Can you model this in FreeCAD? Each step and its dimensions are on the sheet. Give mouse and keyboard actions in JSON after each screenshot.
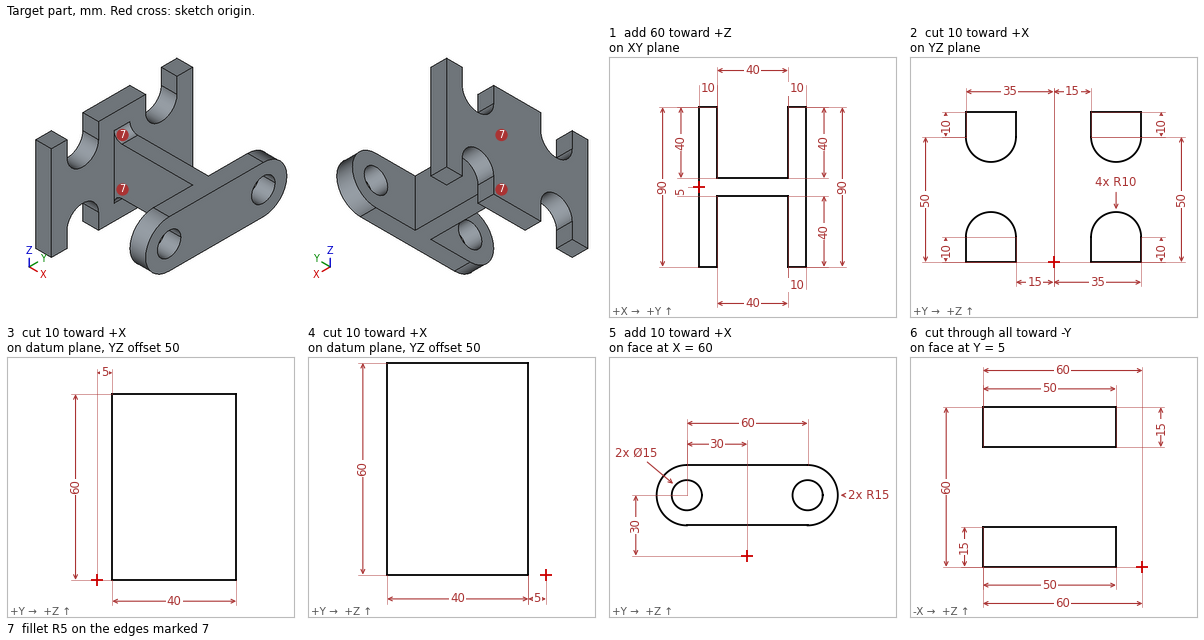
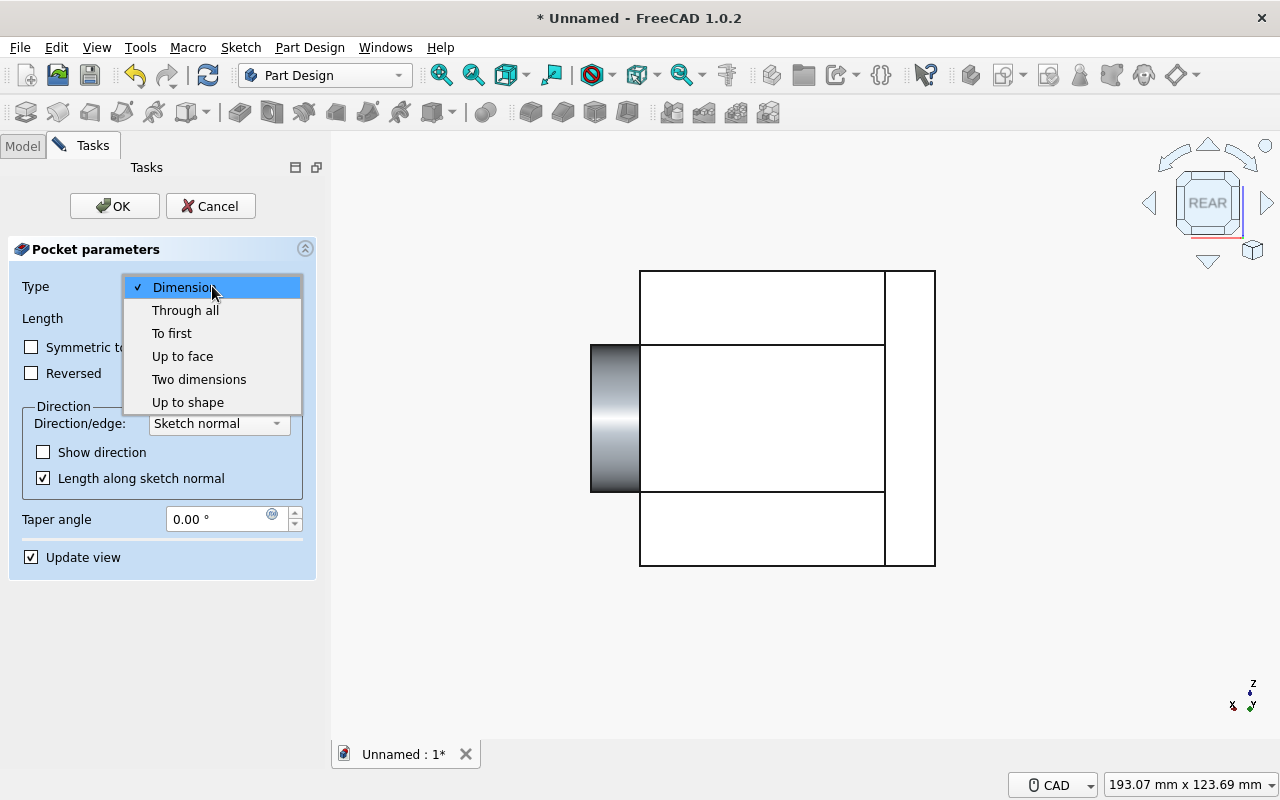
{"action": "left_click", "coordinate": [212, 310]}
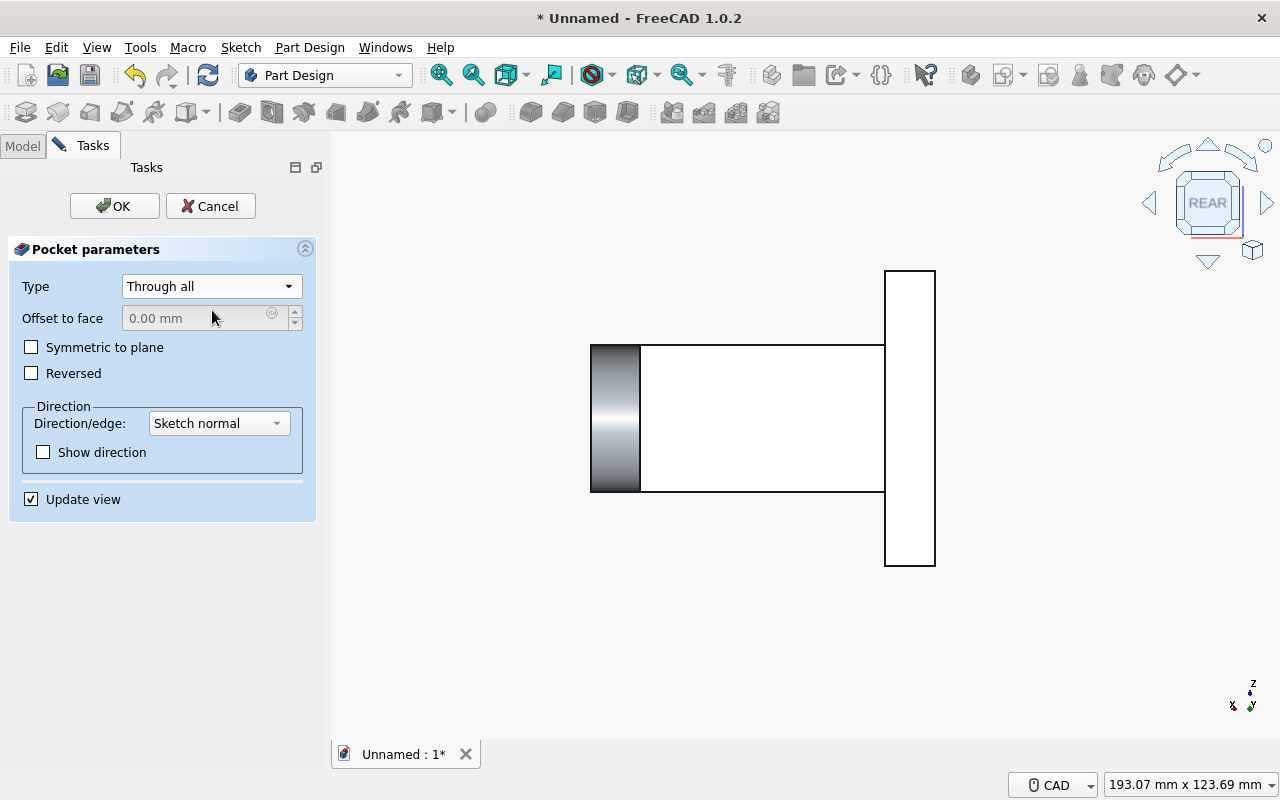
{"action": "left_click", "coordinate": [115, 206]}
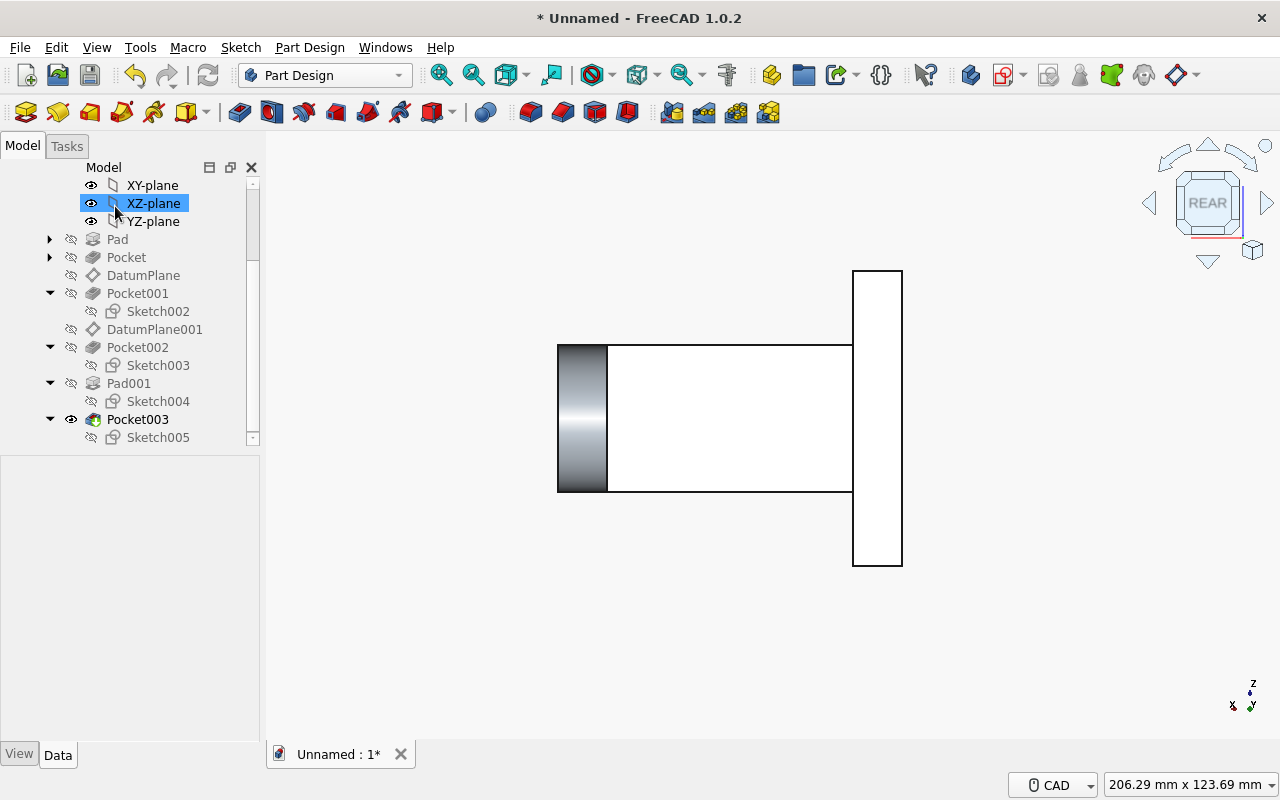
{"action": "key", "text": "0"}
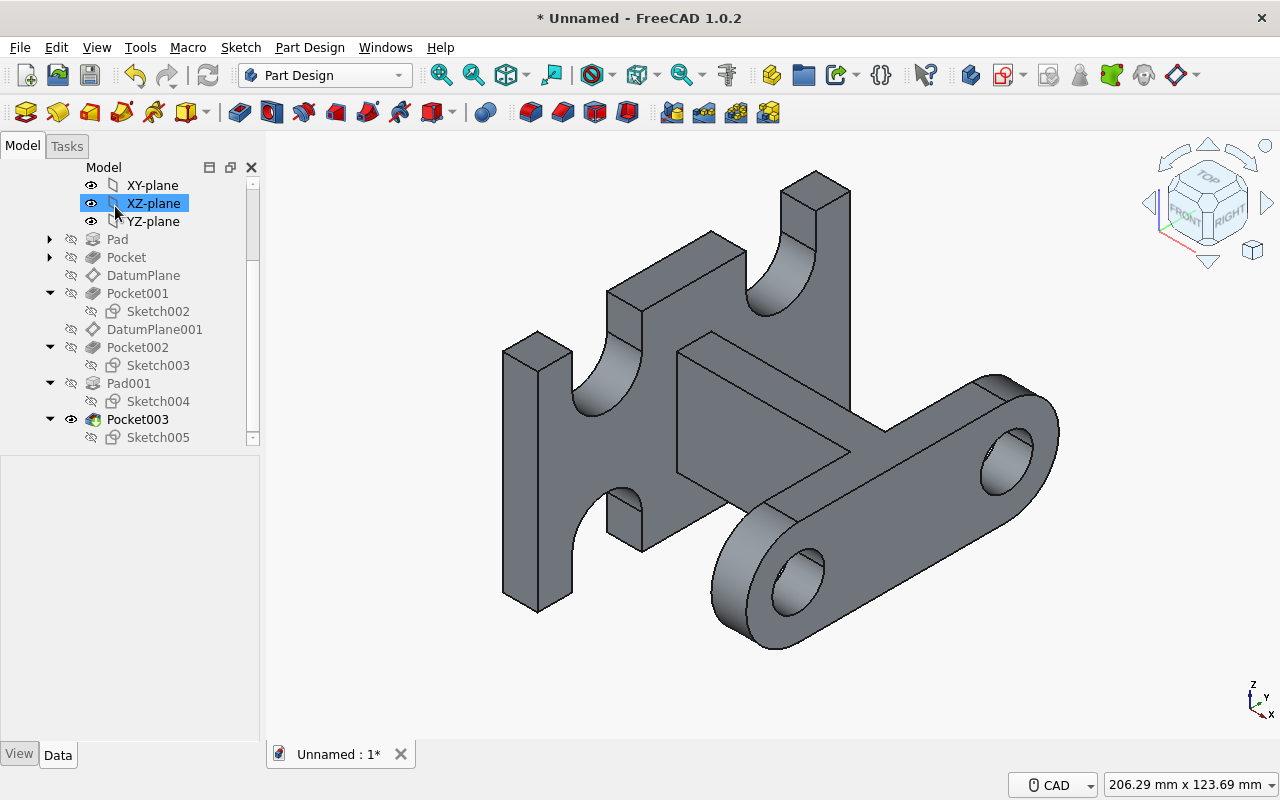
{"action": "key", "text": "2"}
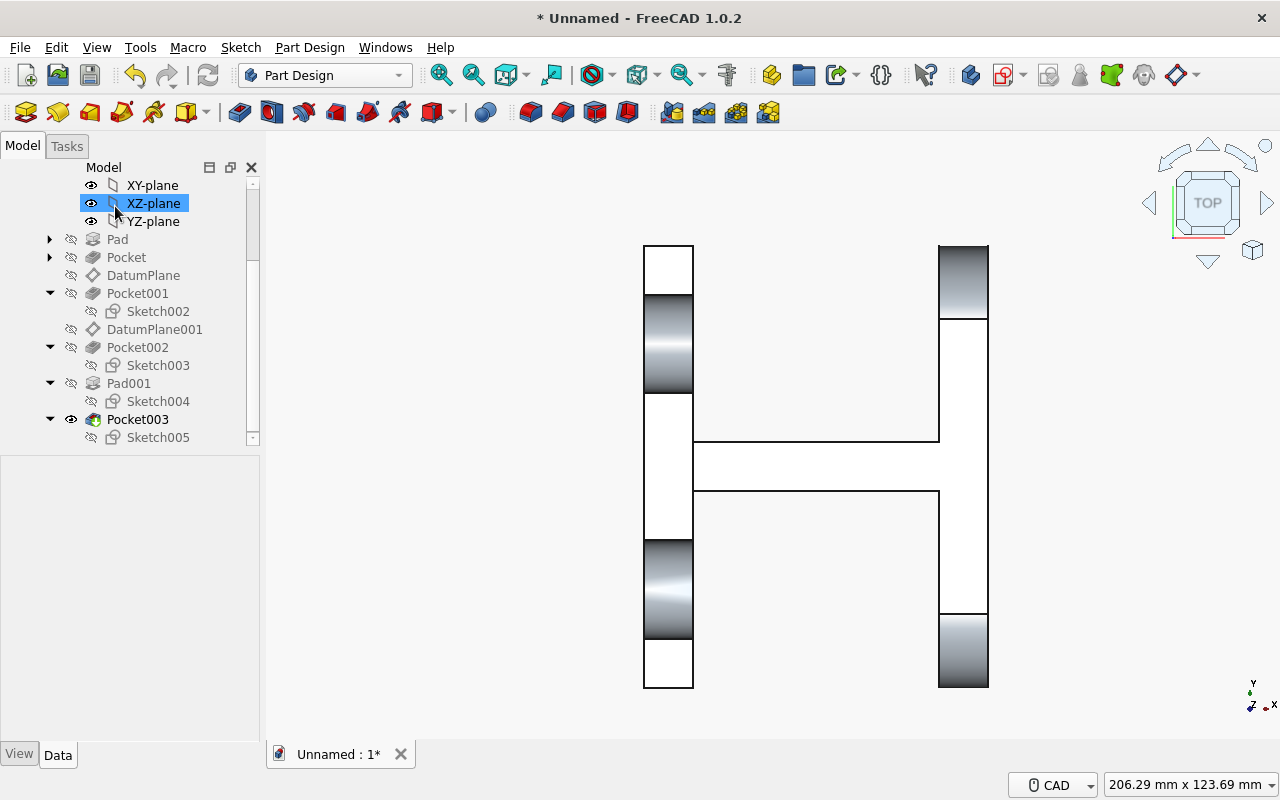
{"action": "key", "text": "1"}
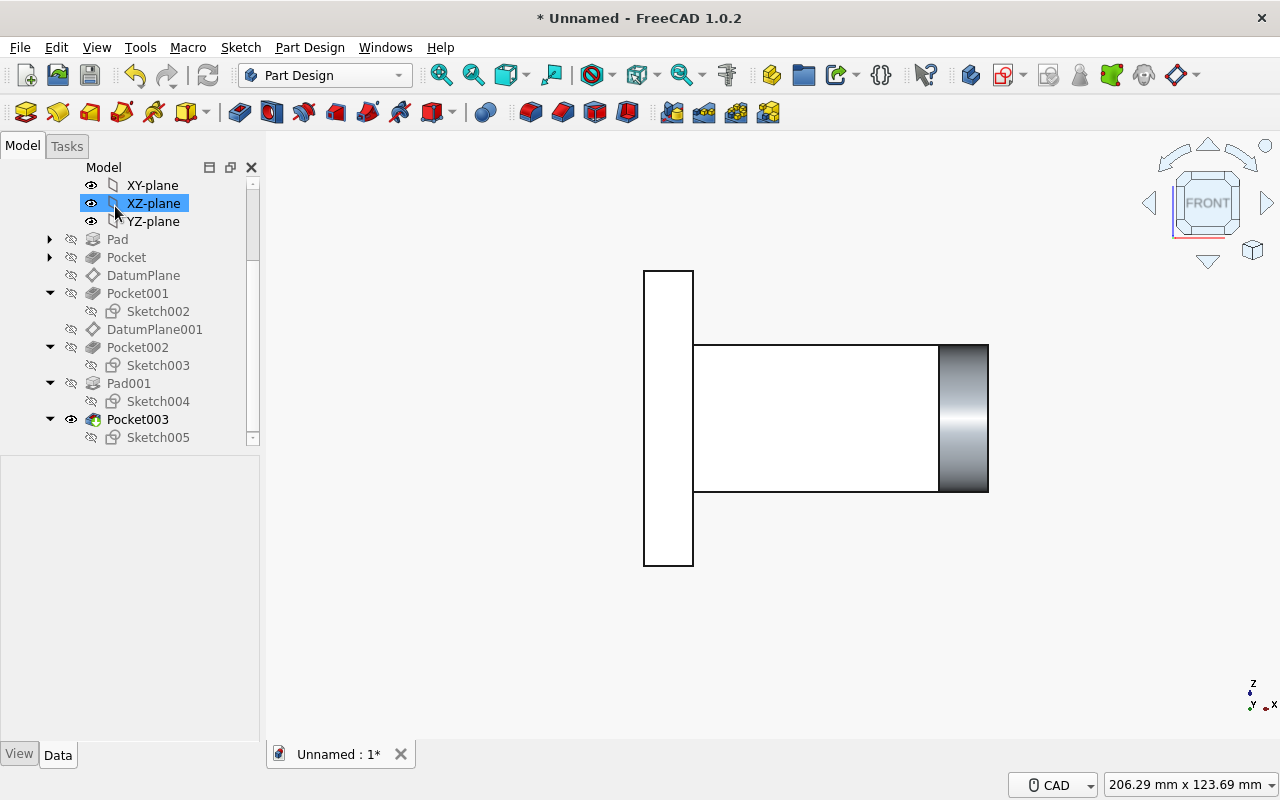
{"action": "key", "text": "3"}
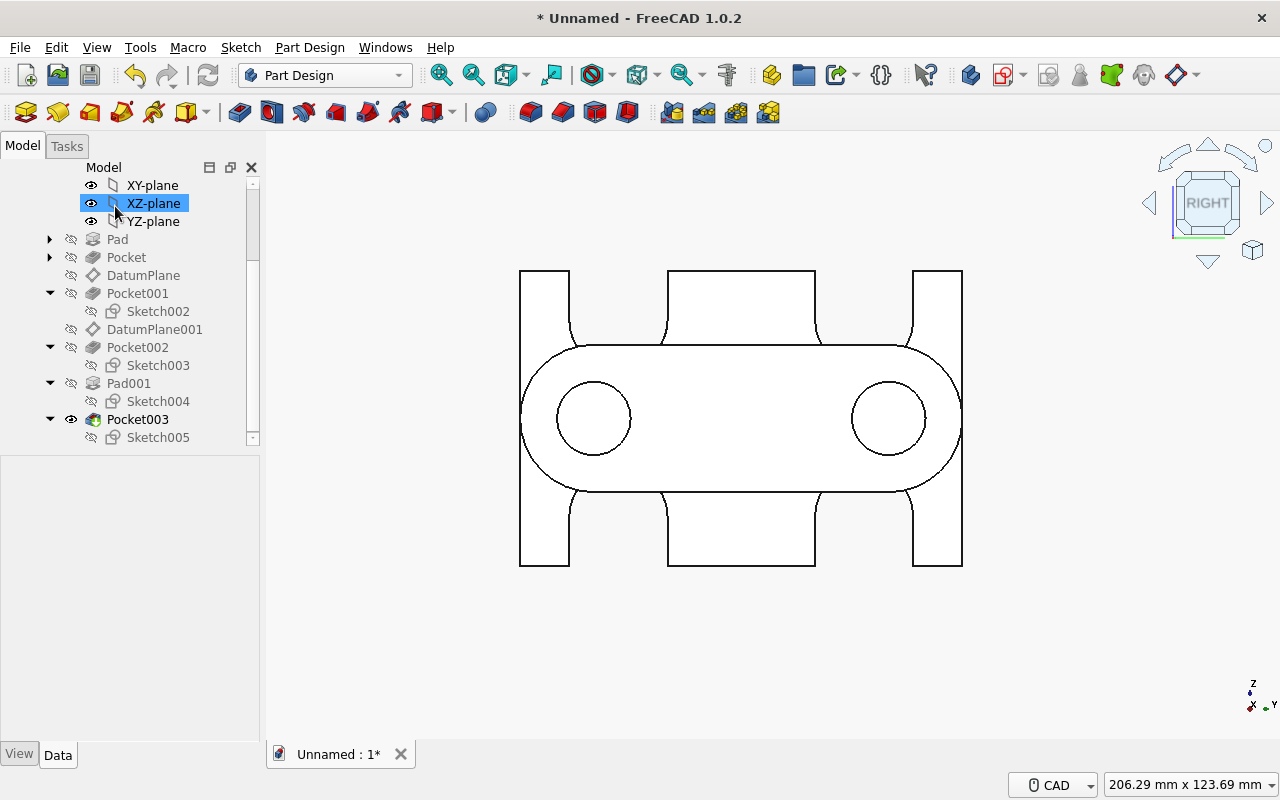
{"action": "key", "text": "5"}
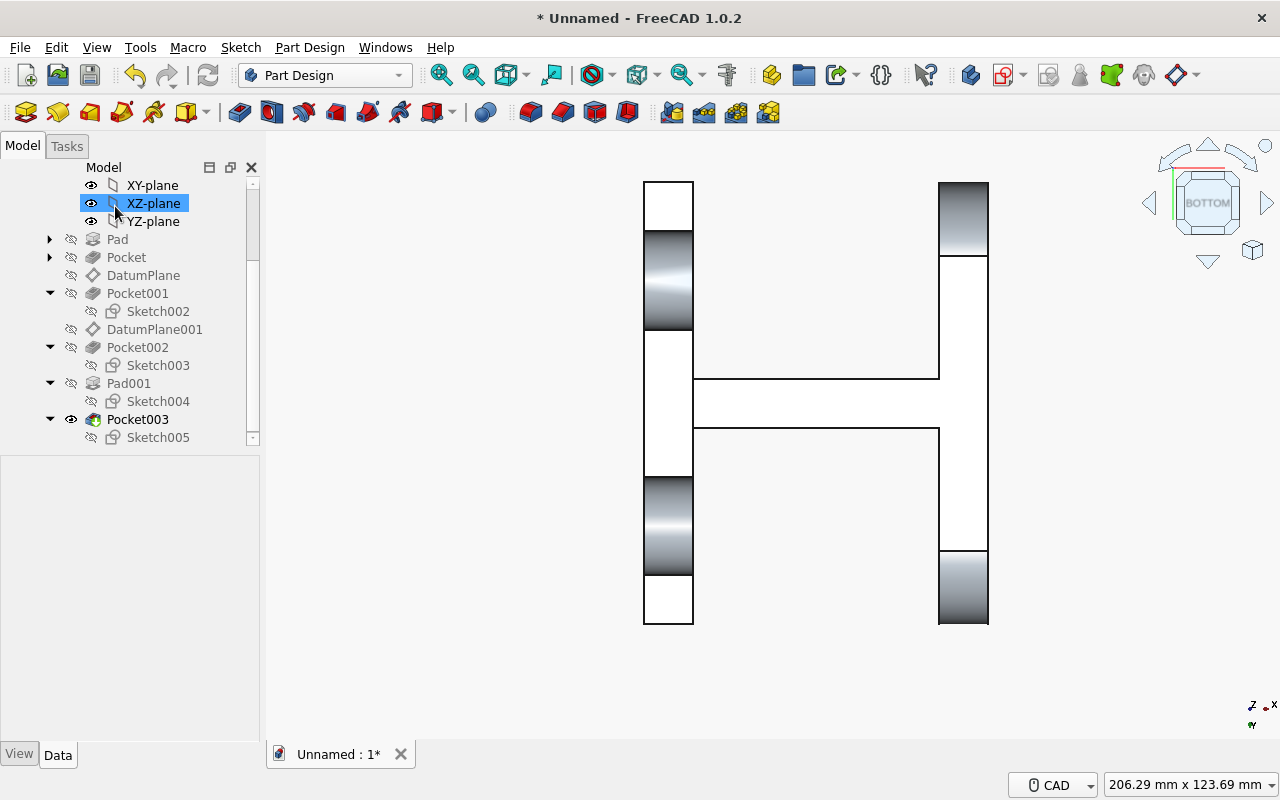
{"action": "key", "text": "4"}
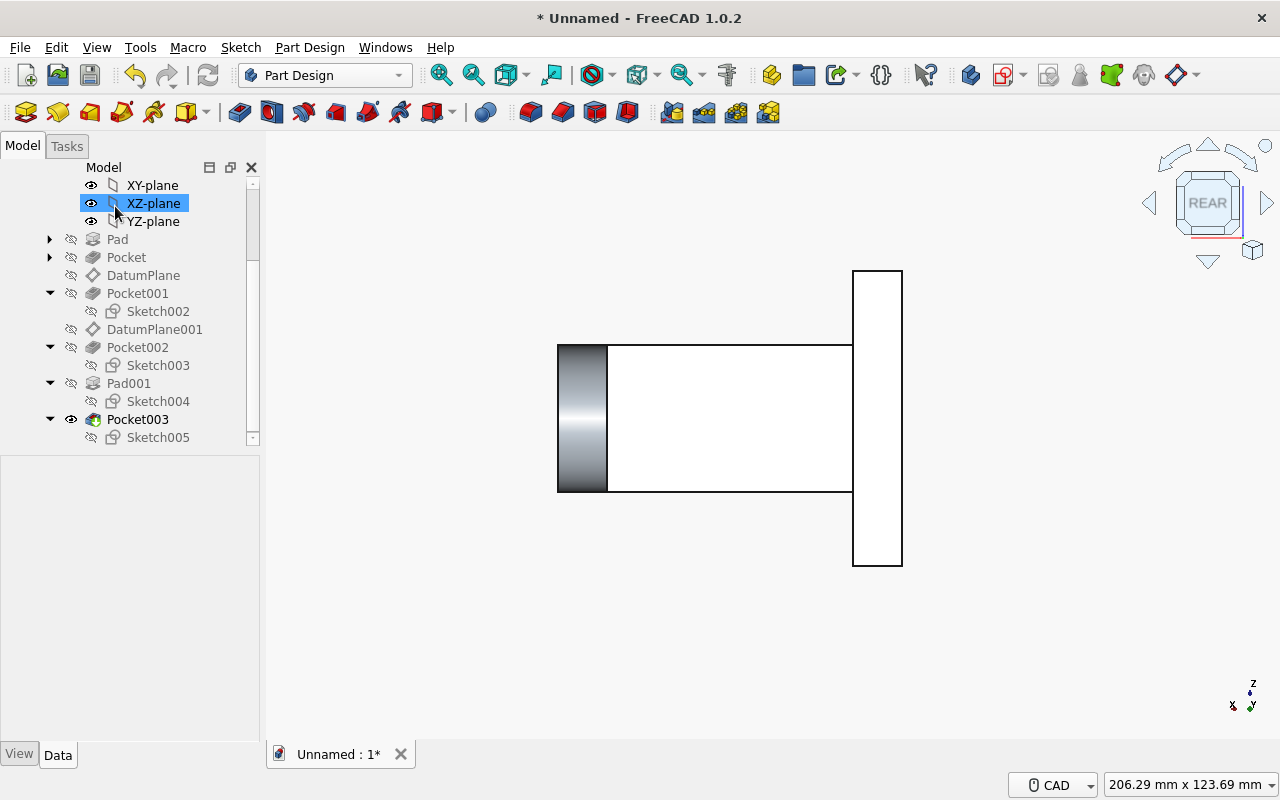
{"action": "key", "text": "6"}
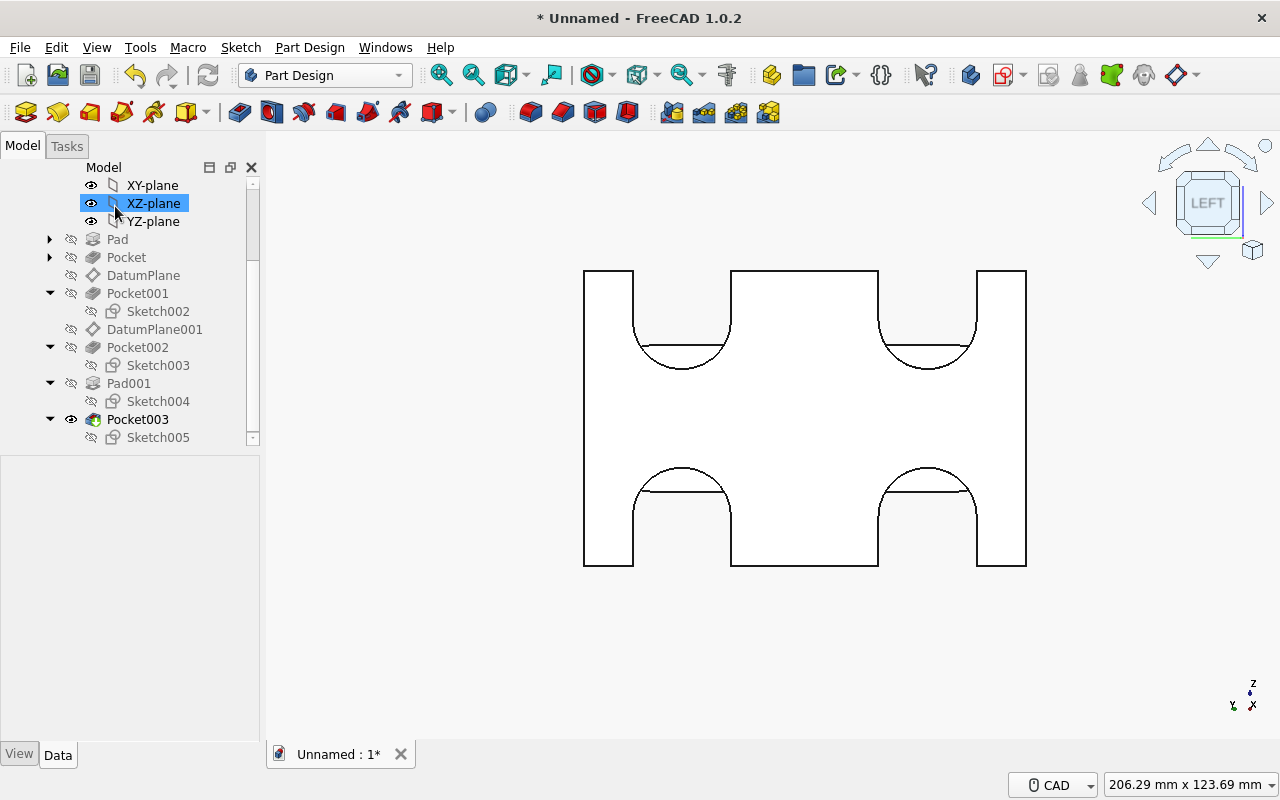
{"action": "key", "text": "v 3"}